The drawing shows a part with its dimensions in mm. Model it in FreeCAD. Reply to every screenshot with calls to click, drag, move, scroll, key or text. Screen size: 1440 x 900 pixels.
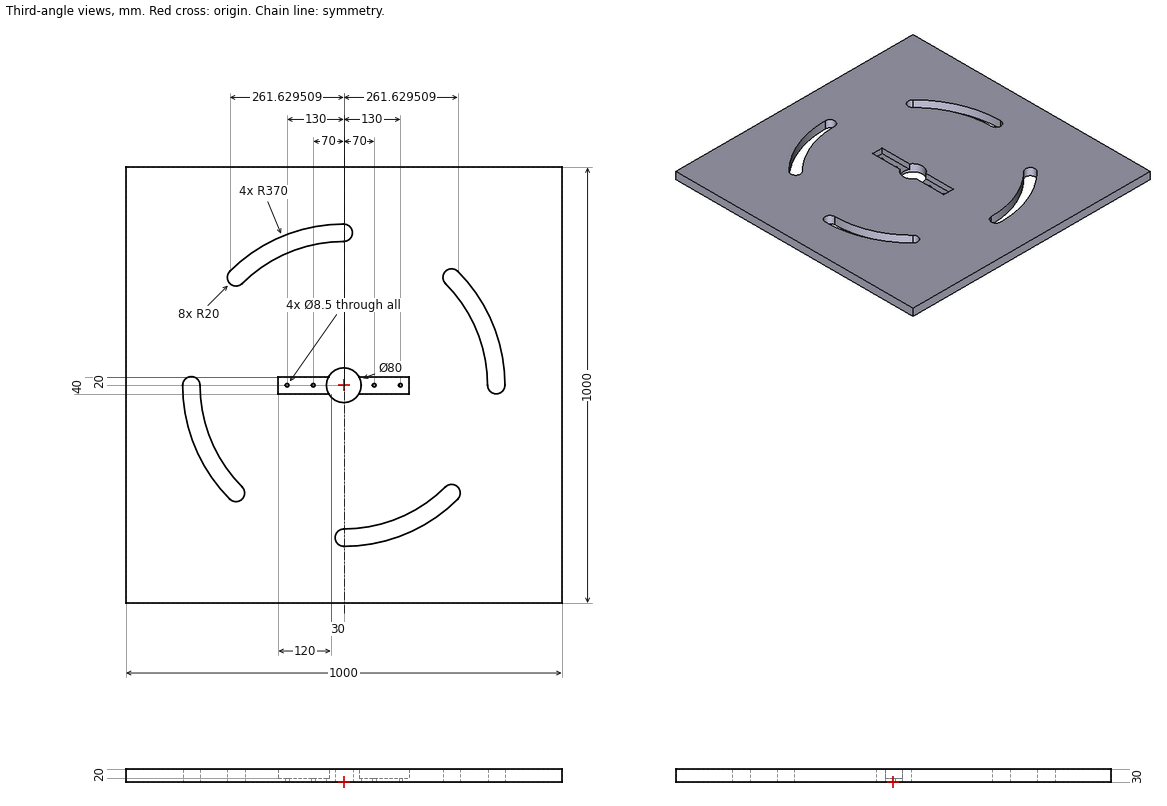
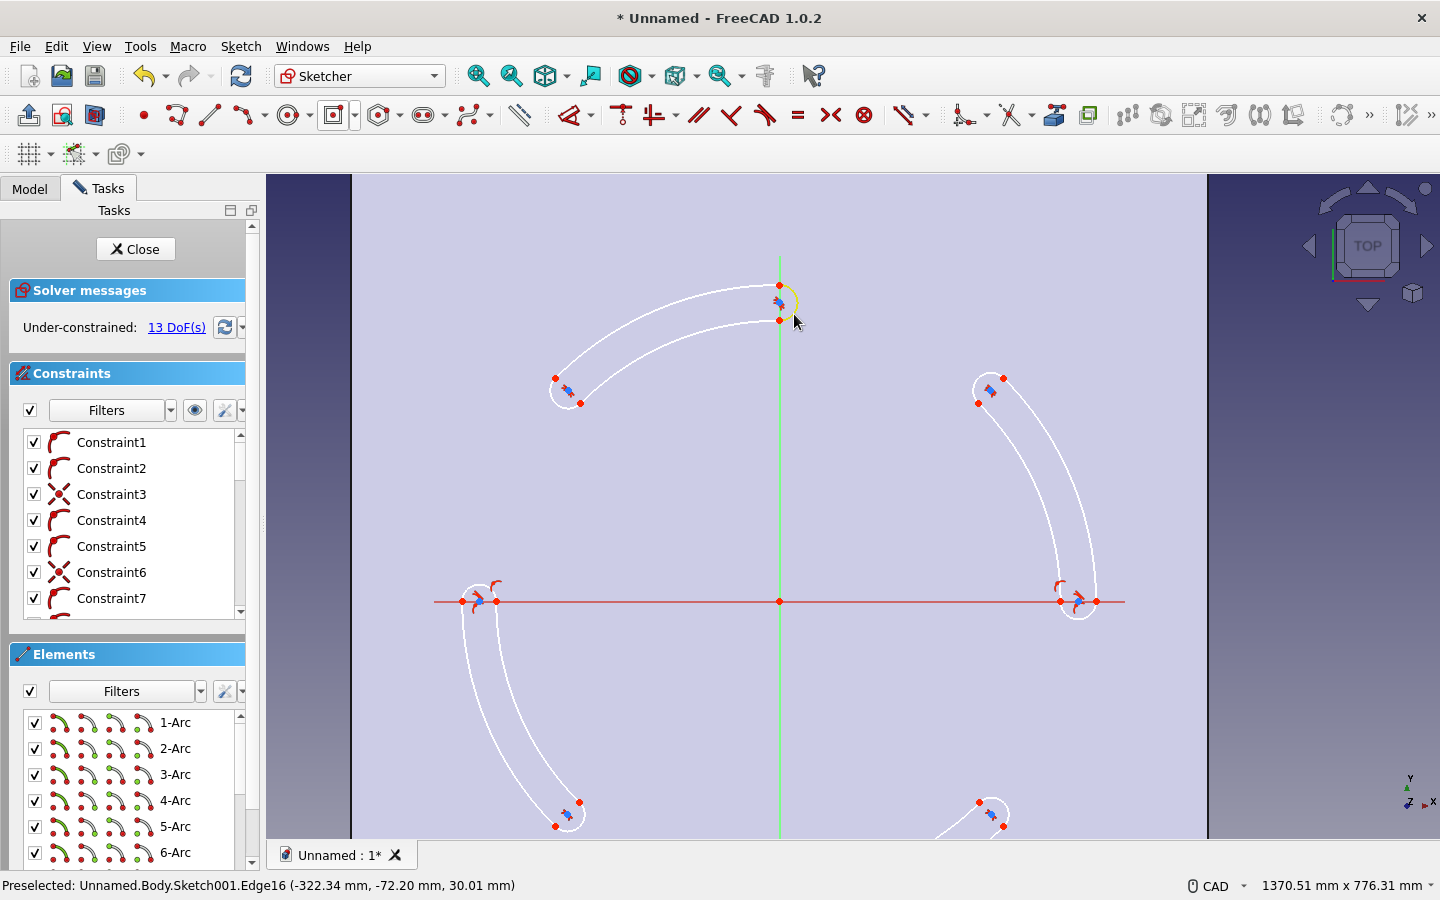
click(794, 313)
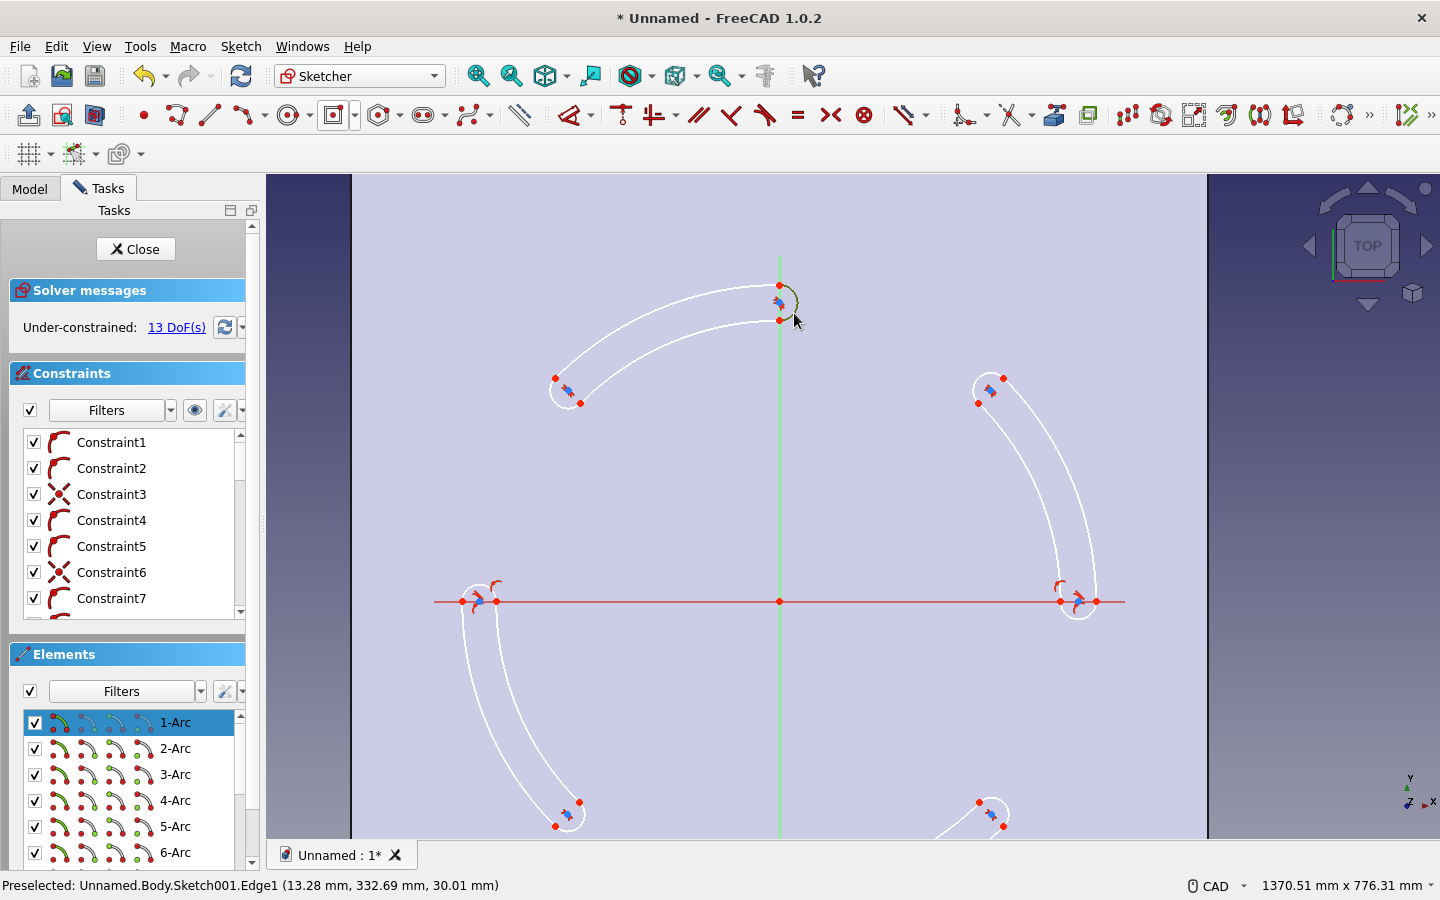
click(1068, 616)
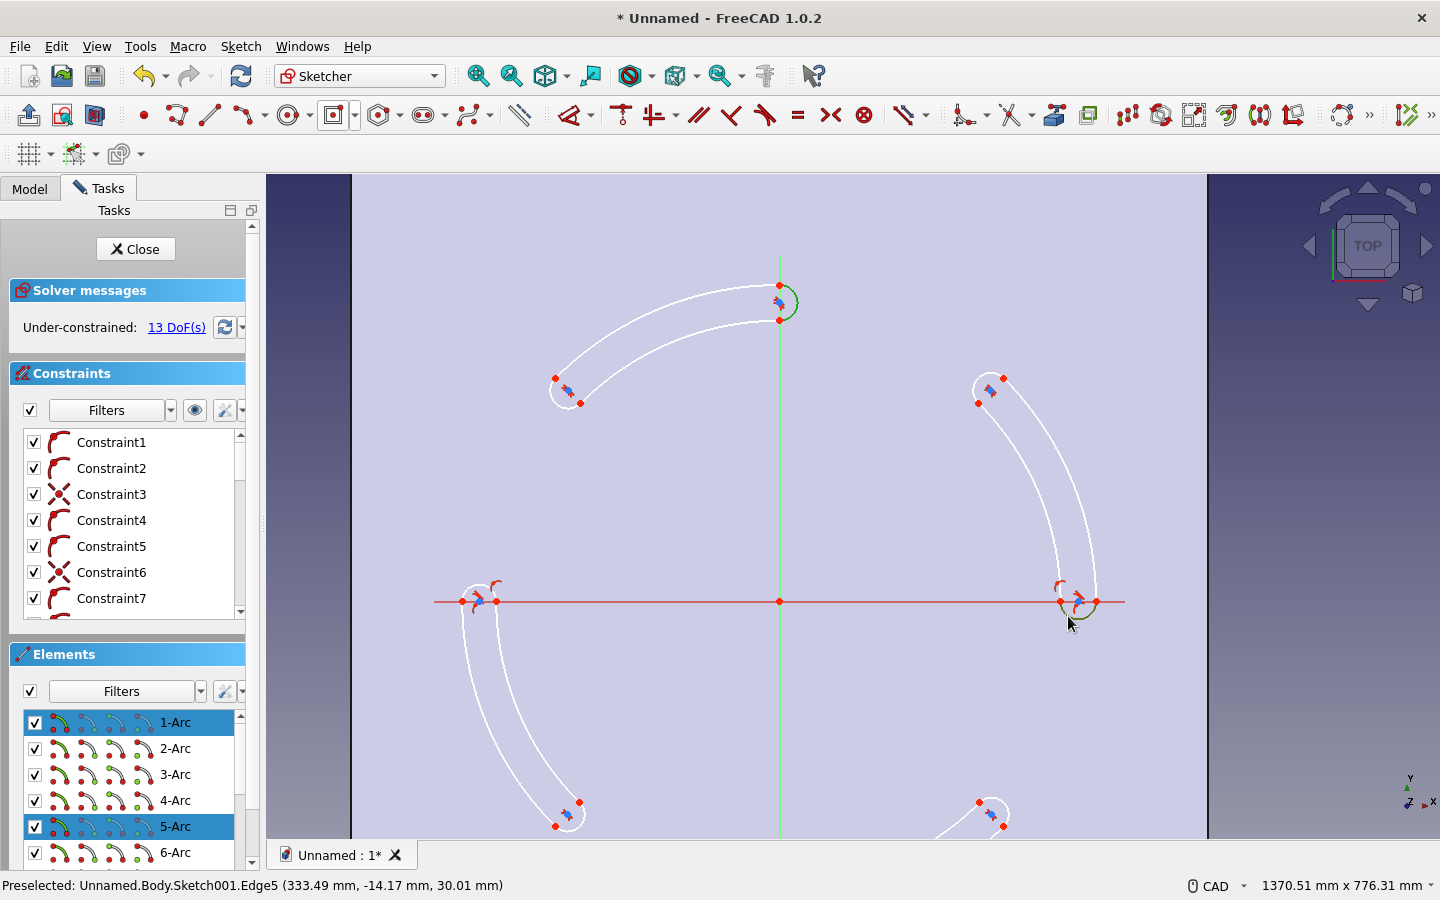
scroll(794, 313, down, 2)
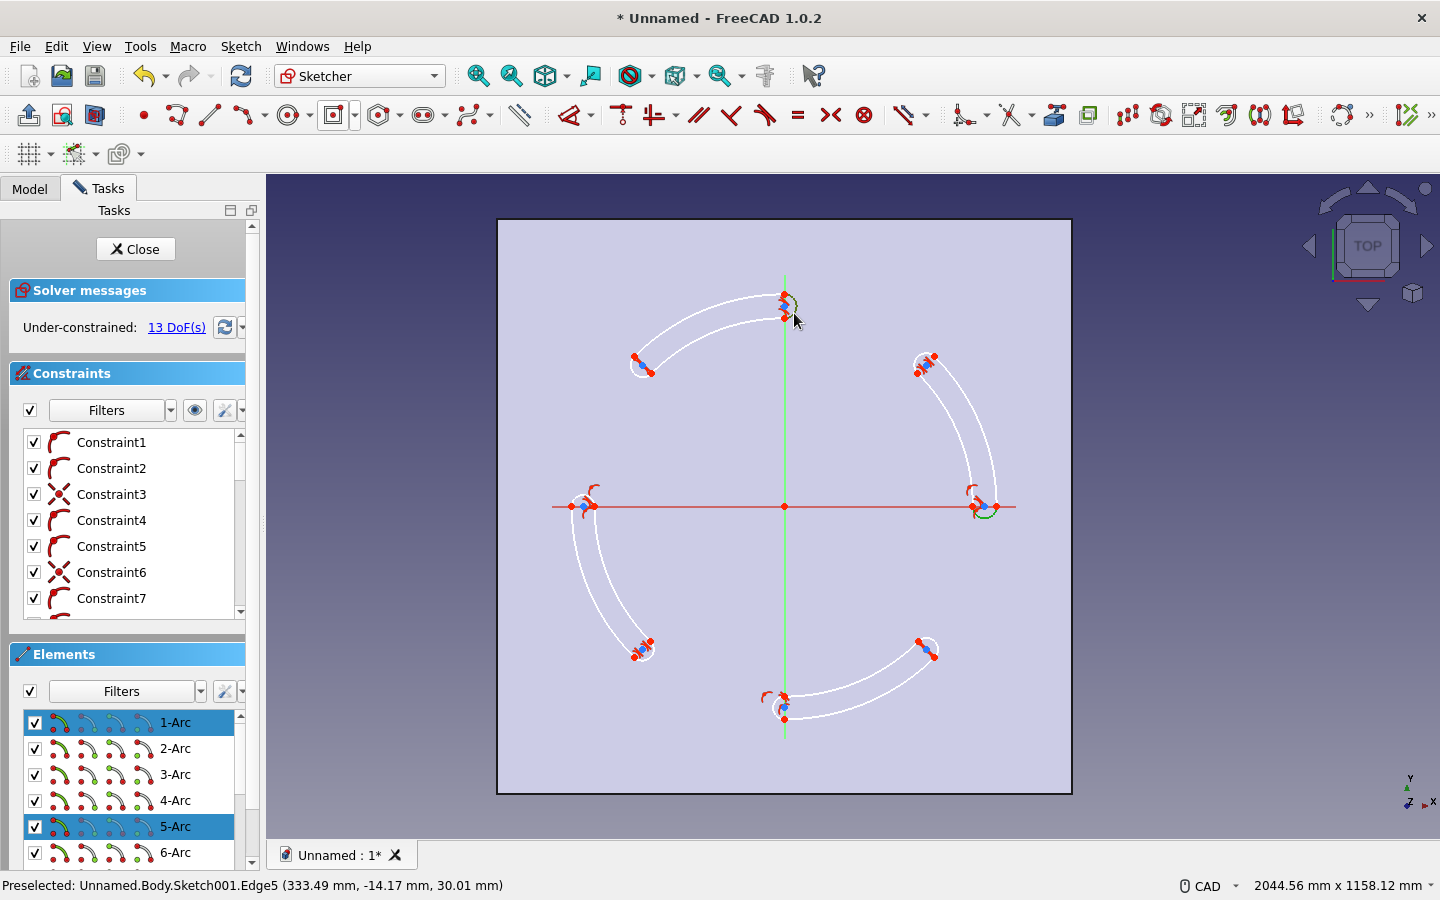
scroll(775, 701, up, 3)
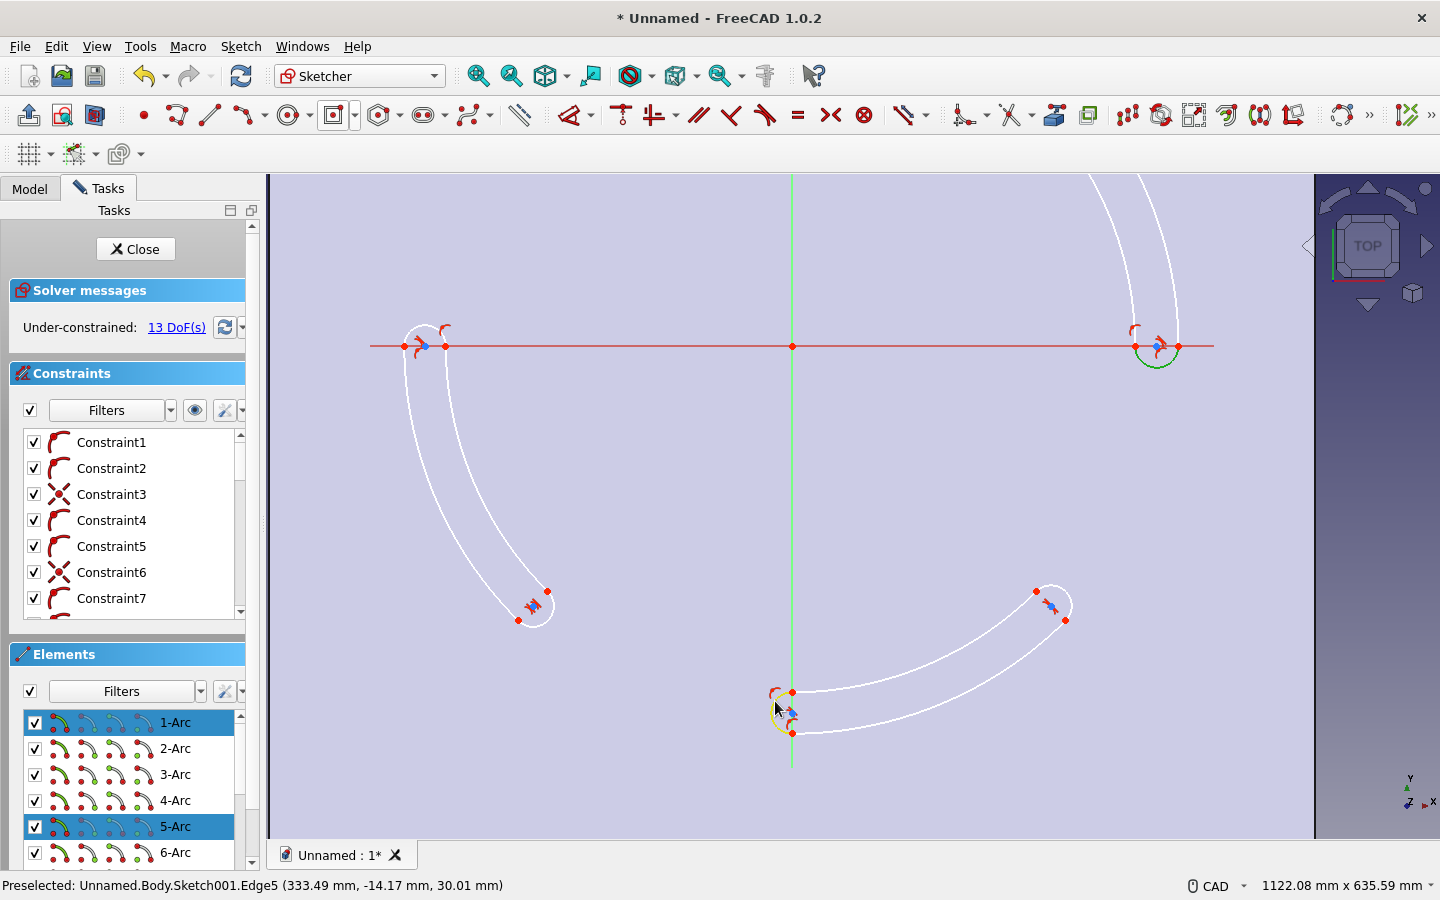
click(775, 701)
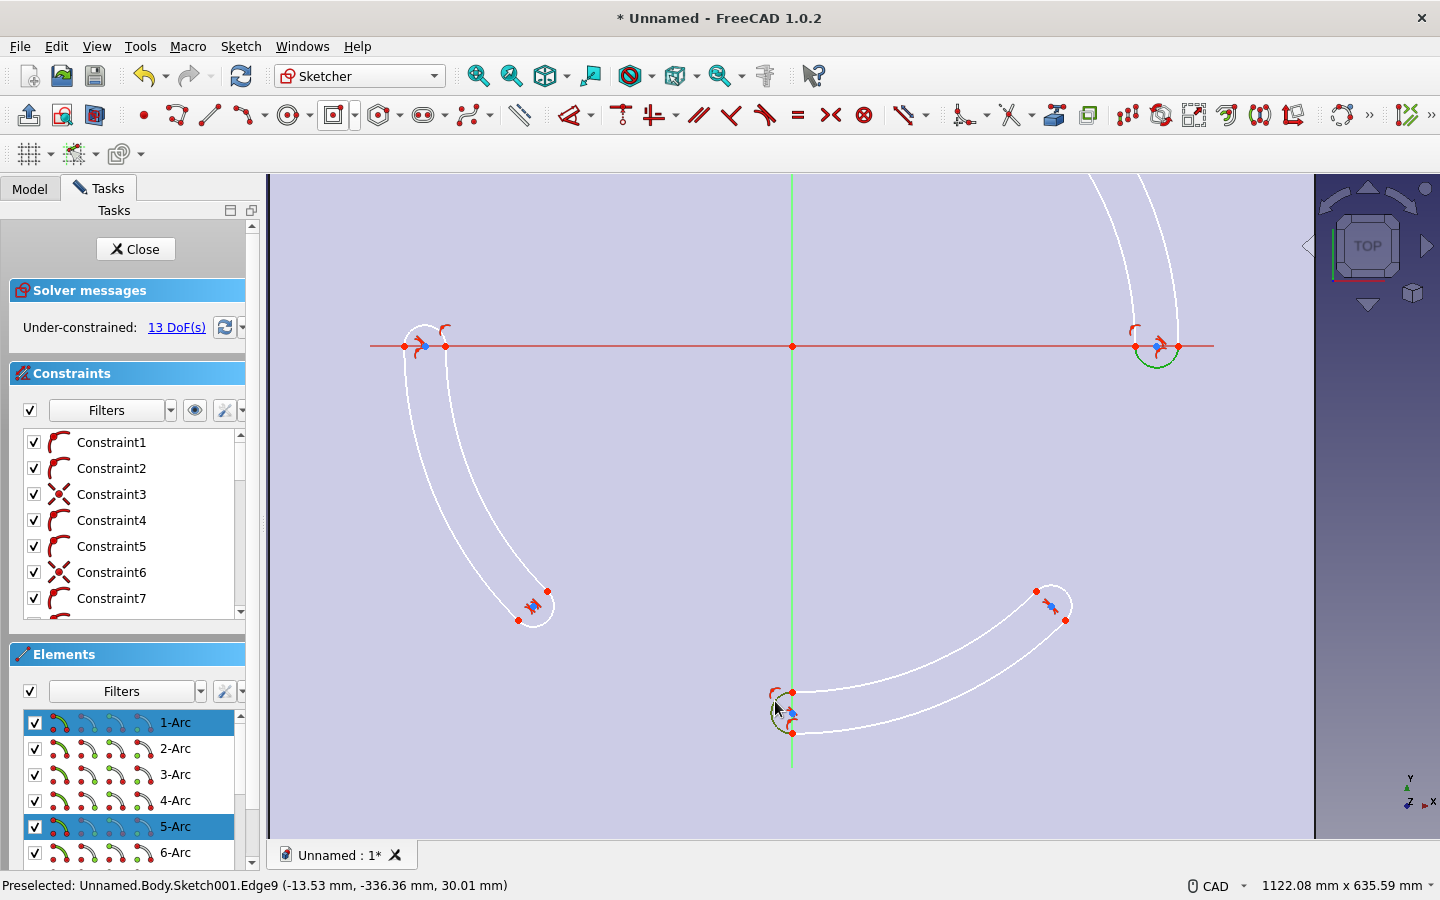
click(437, 329)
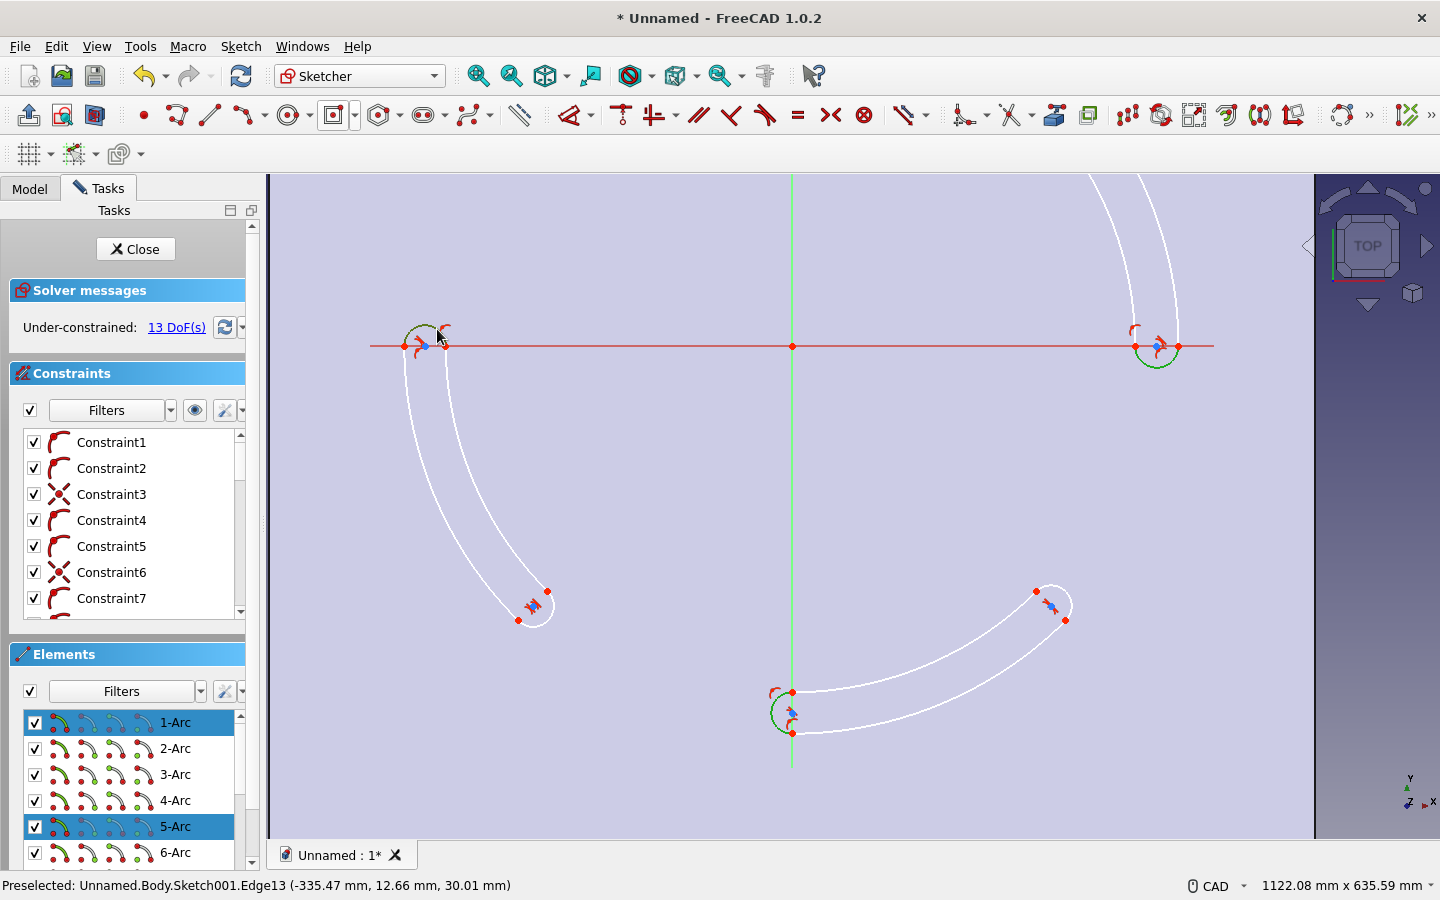
click(798, 116)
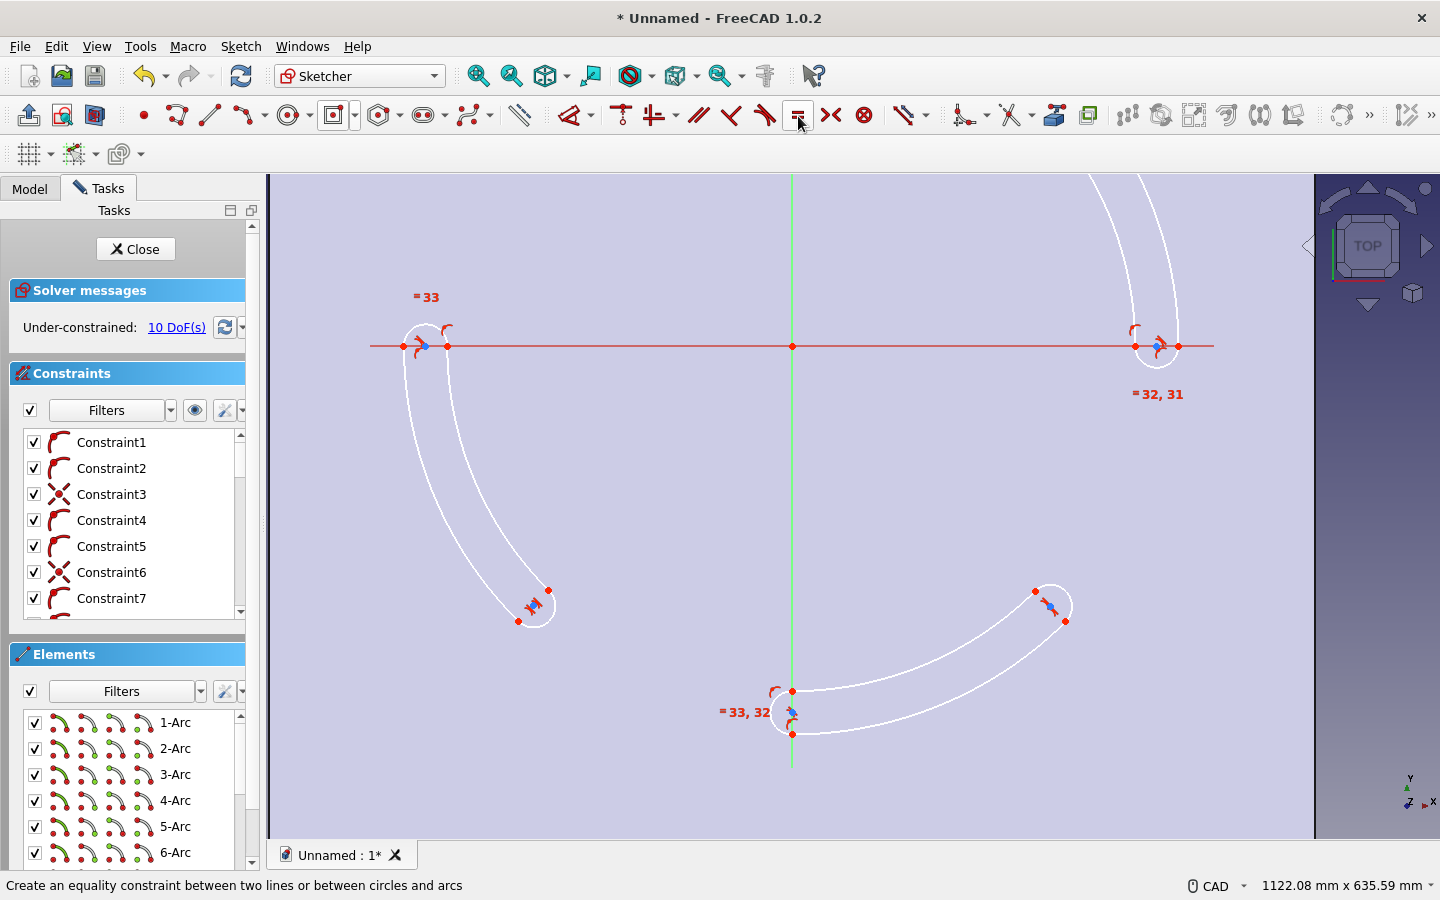
scroll(775, 702, down, 3)